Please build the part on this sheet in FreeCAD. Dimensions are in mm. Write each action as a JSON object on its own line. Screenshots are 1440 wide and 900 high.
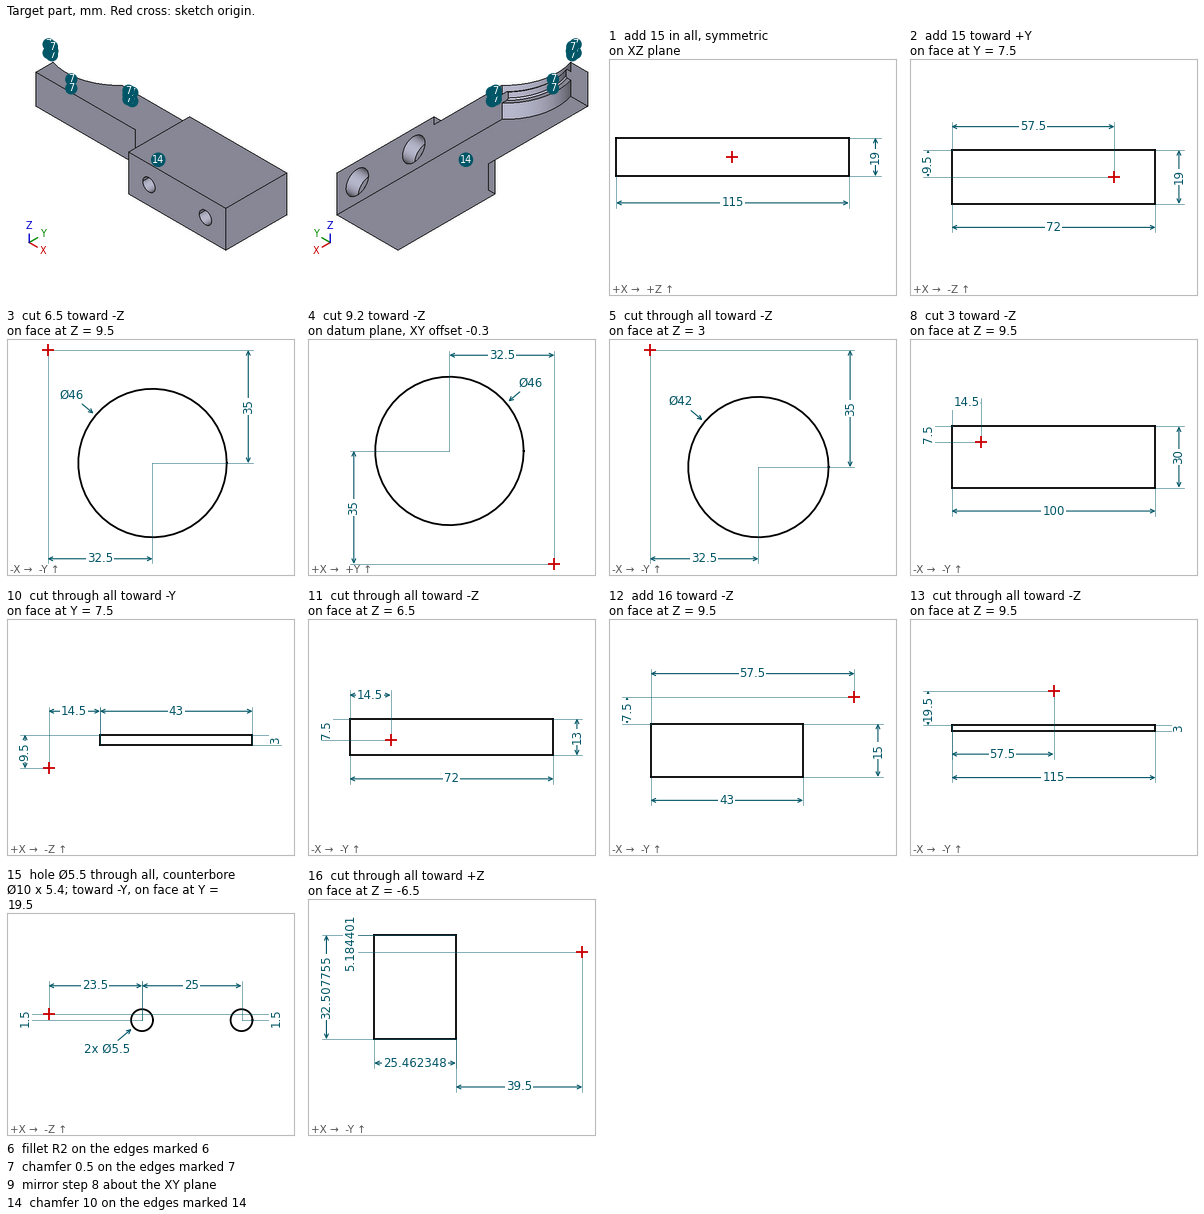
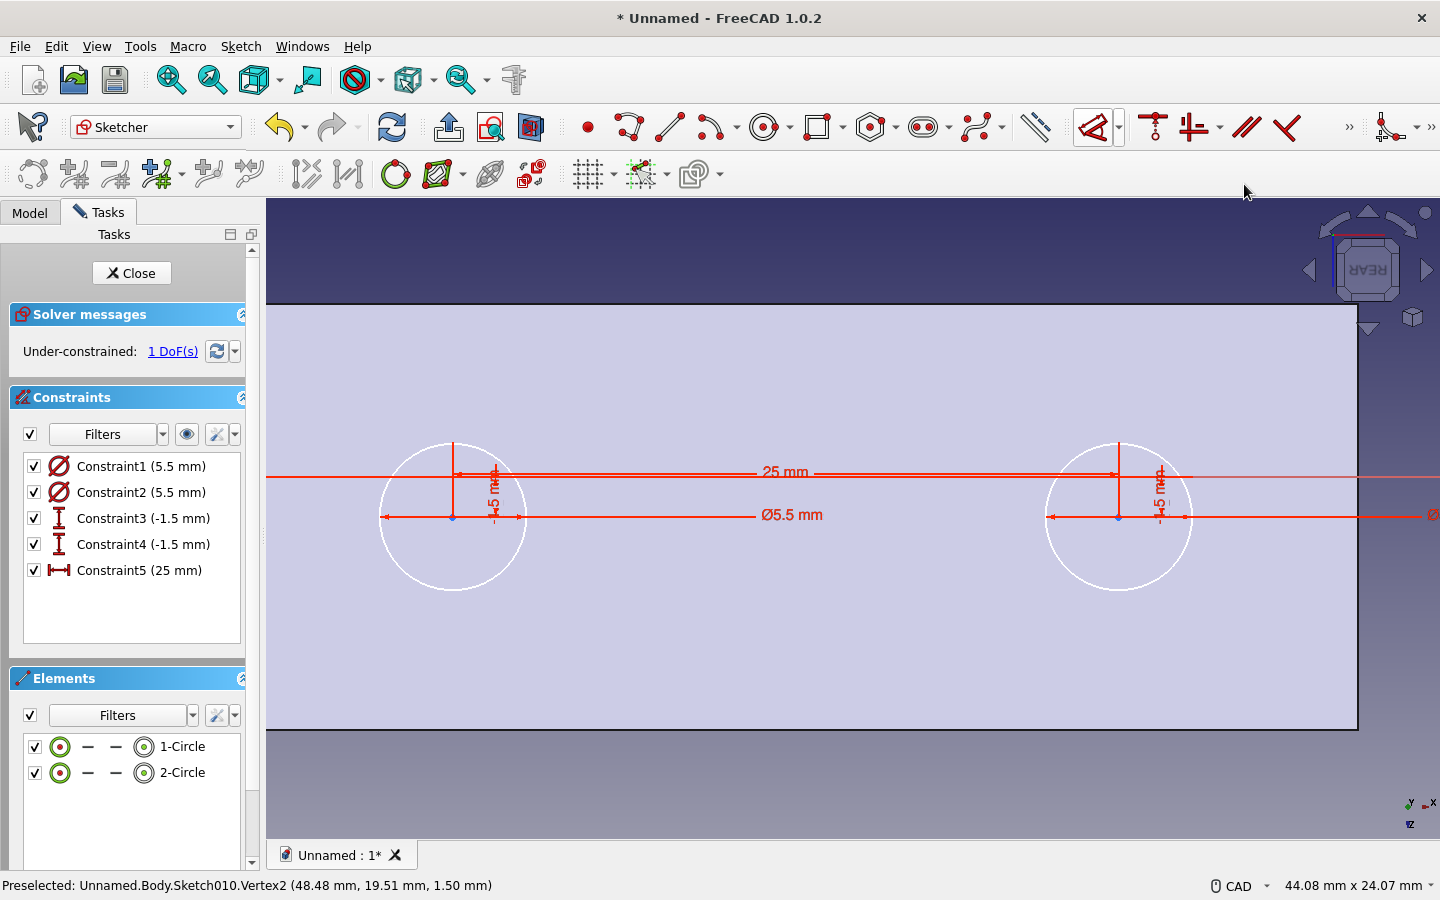
{"action": "left_click", "coordinate": [453, 517]}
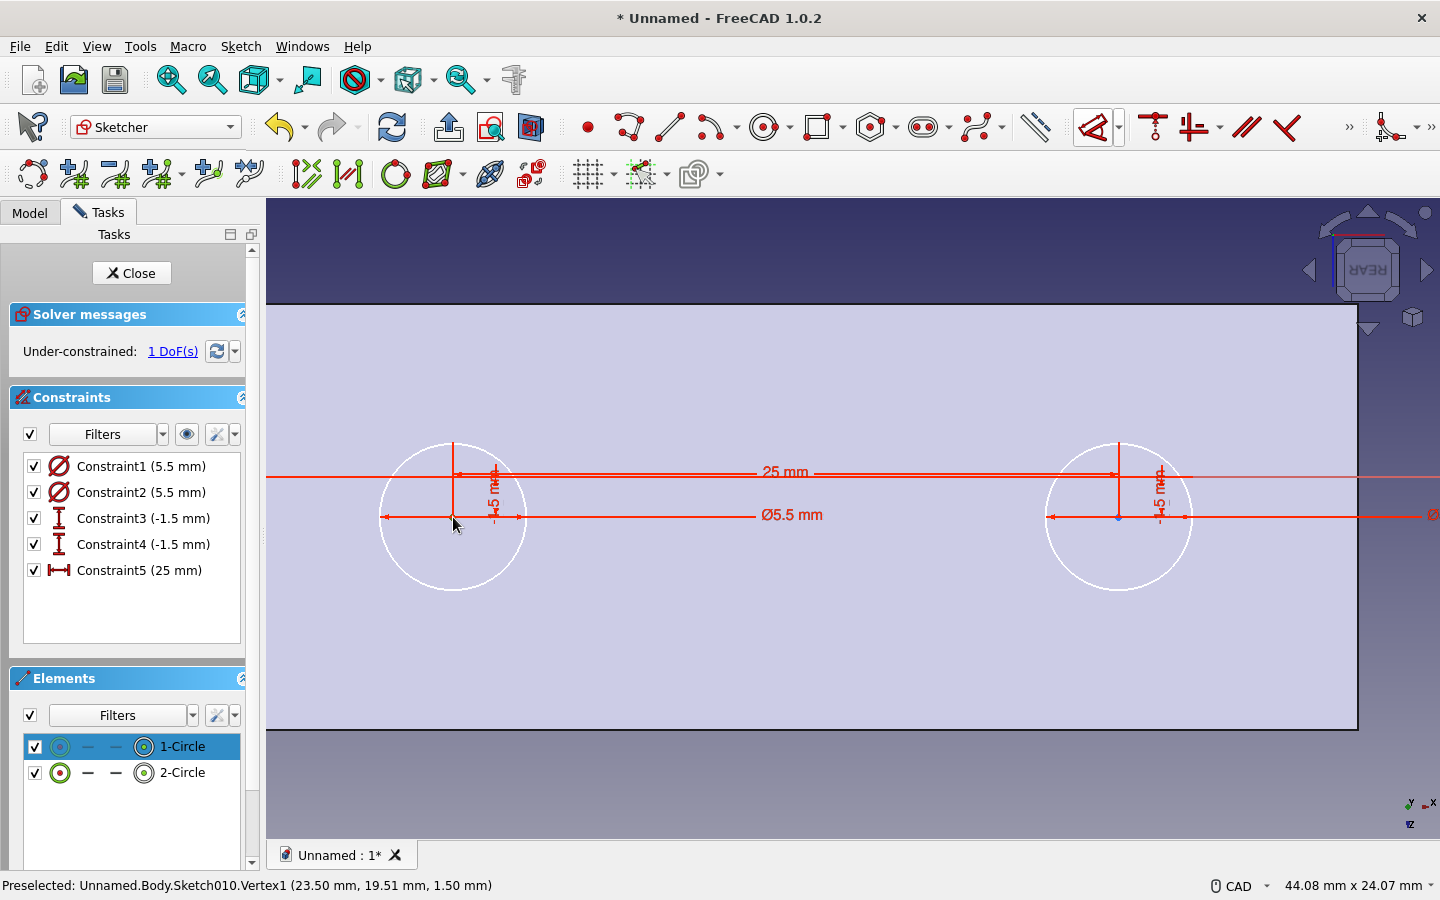
{"action": "left_click", "coordinate": [1118, 128]}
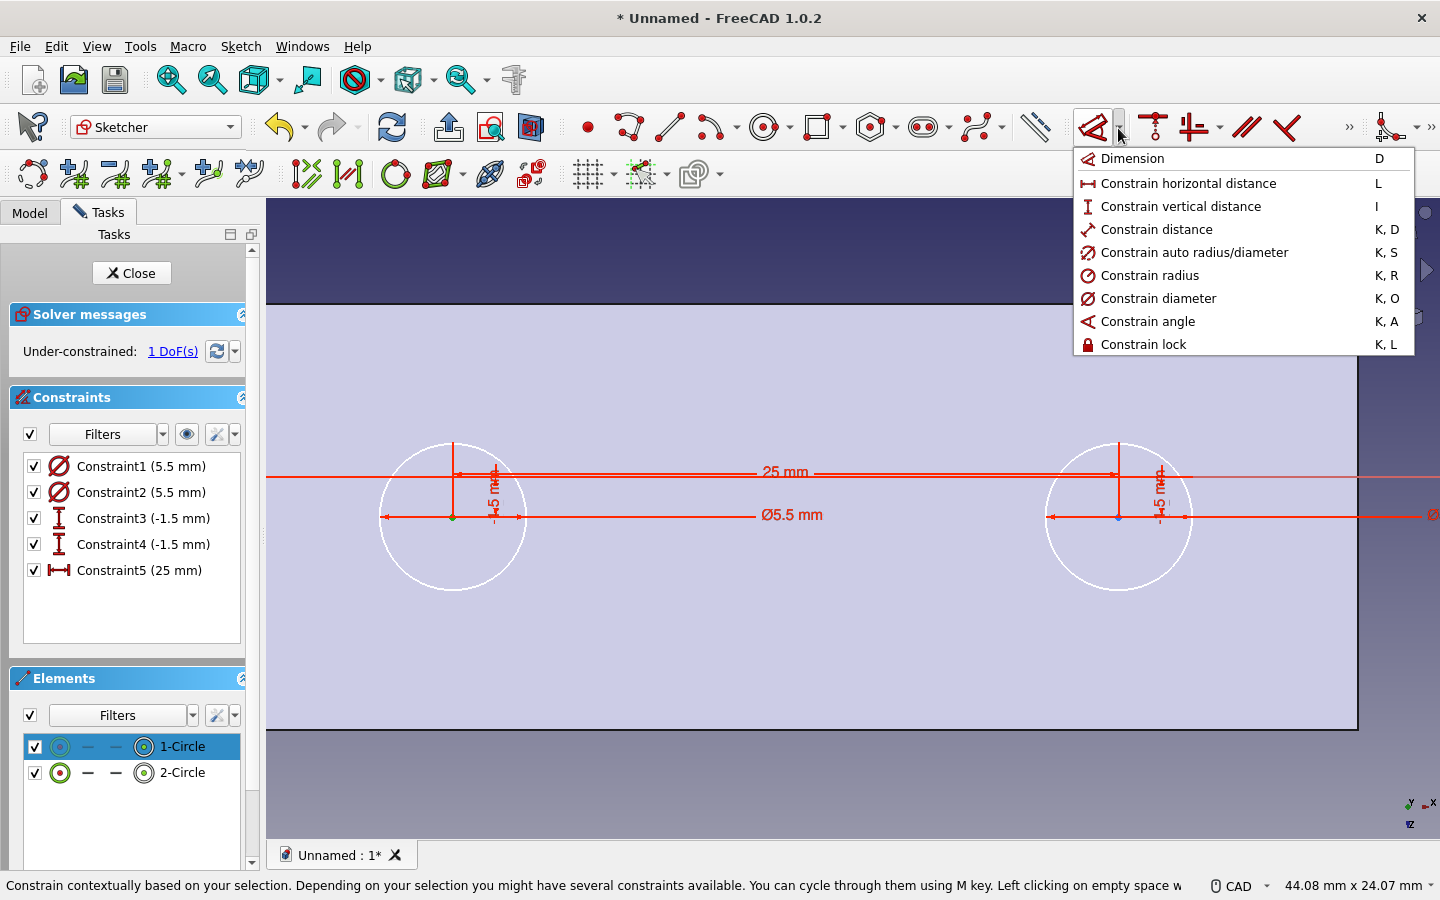
{"action": "left_click", "coordinate": [1244, 184]}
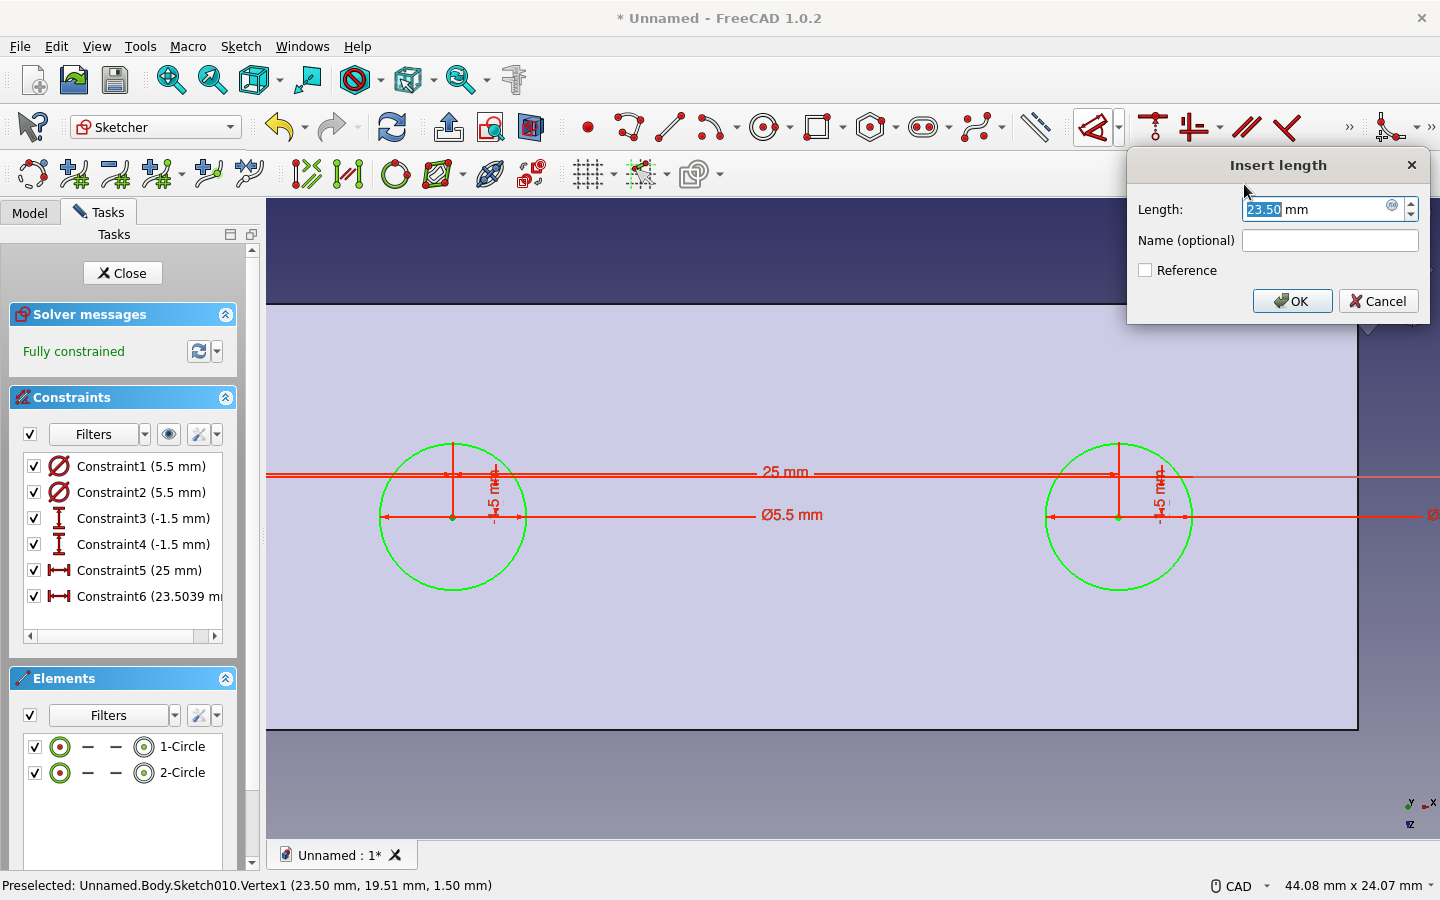
{"action": "type", "text": "23.5"}
{"action": "key", "text": "Return"}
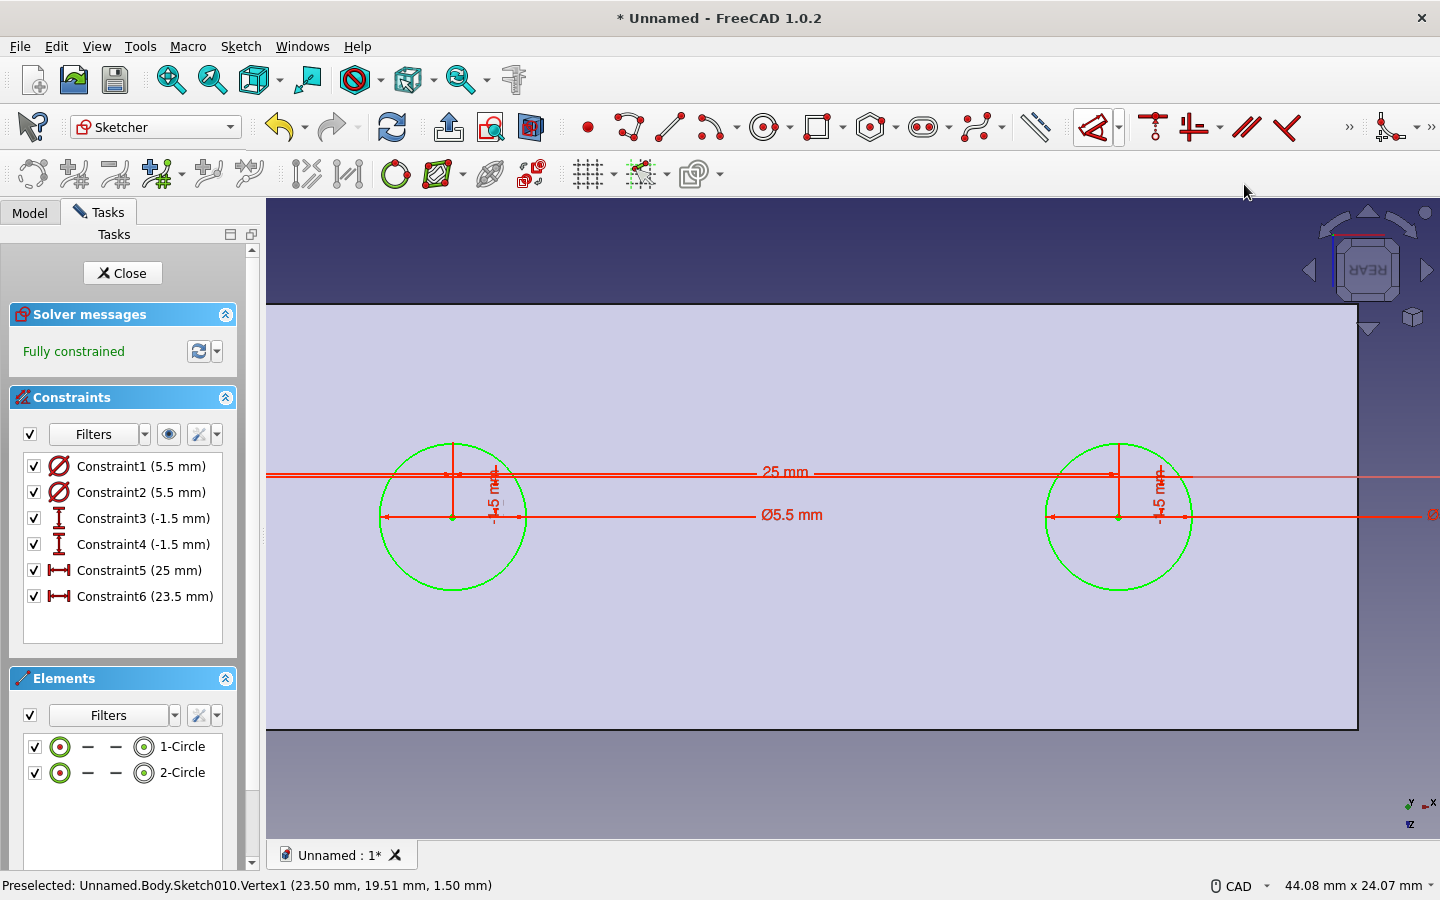
{"action": "left_click", "coordinate": [123, 273]}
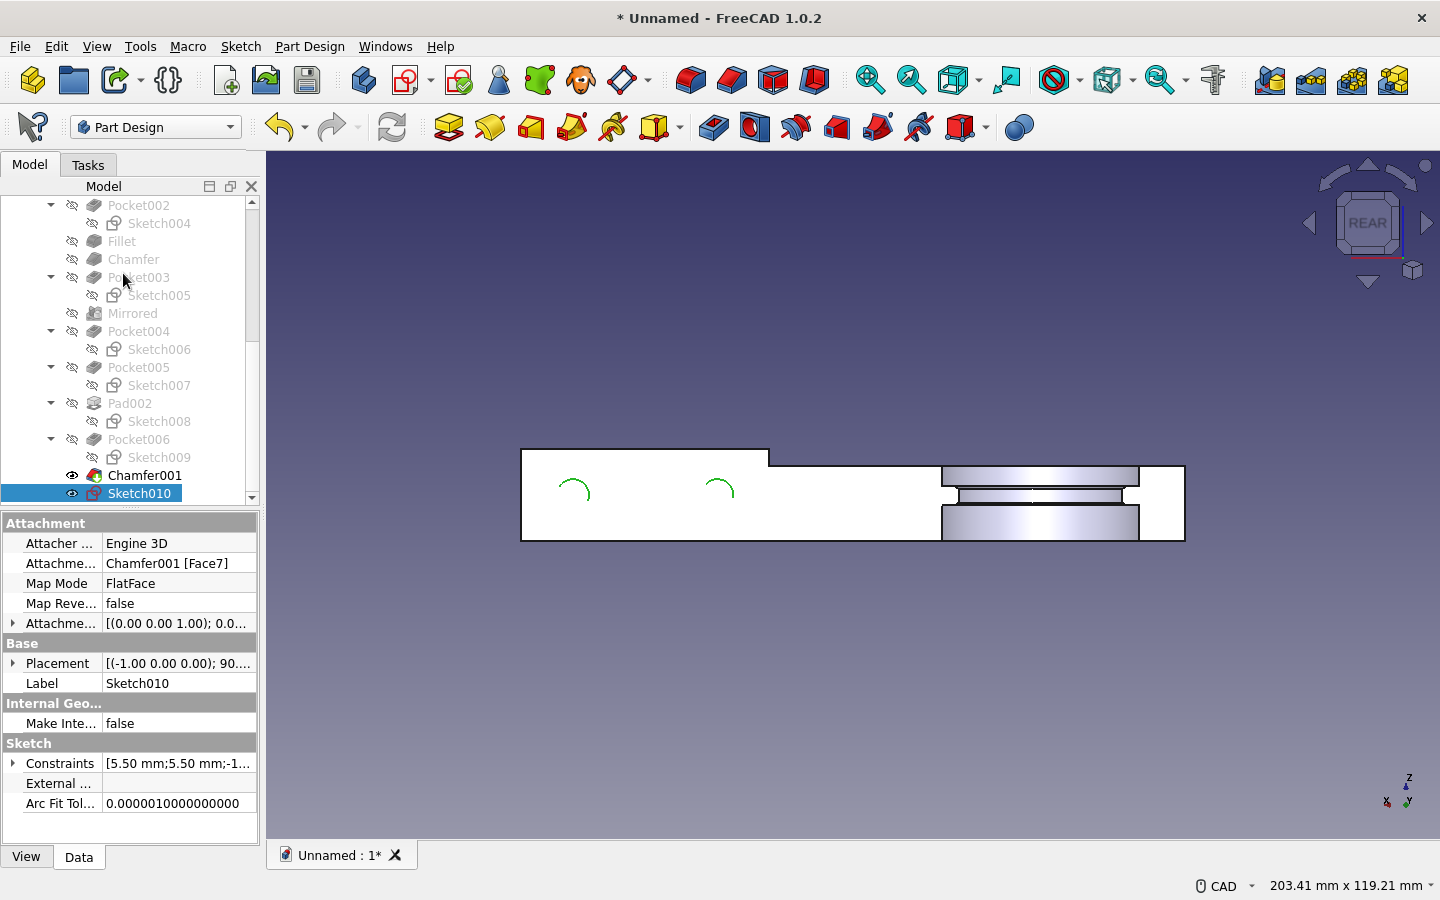
{"action": "left_click", "coordinate": [755, 128]}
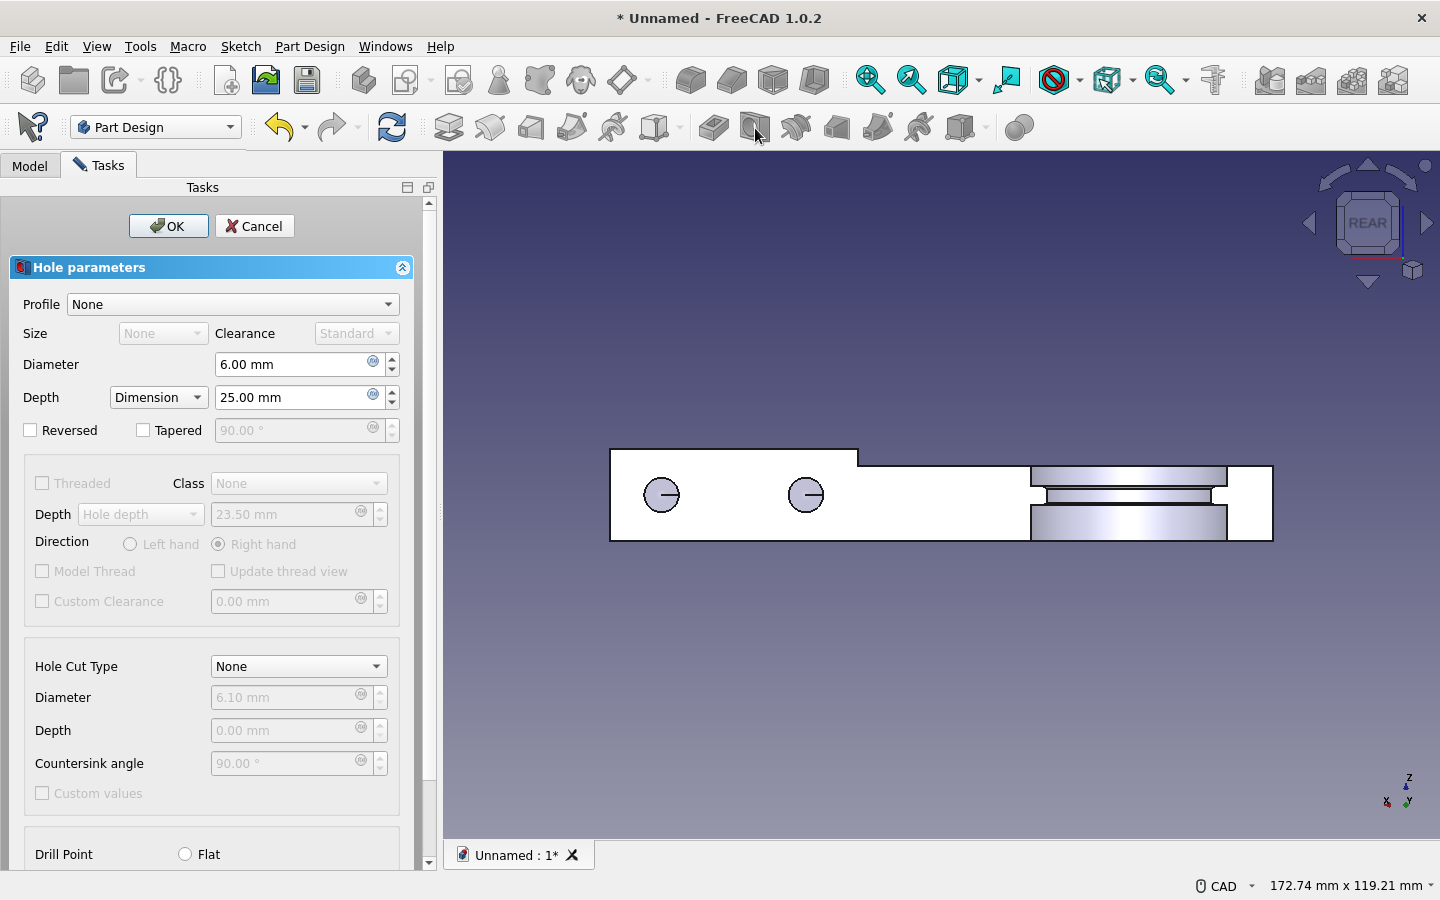
{"action": "triple_click", "coordinate": [300, 364]}